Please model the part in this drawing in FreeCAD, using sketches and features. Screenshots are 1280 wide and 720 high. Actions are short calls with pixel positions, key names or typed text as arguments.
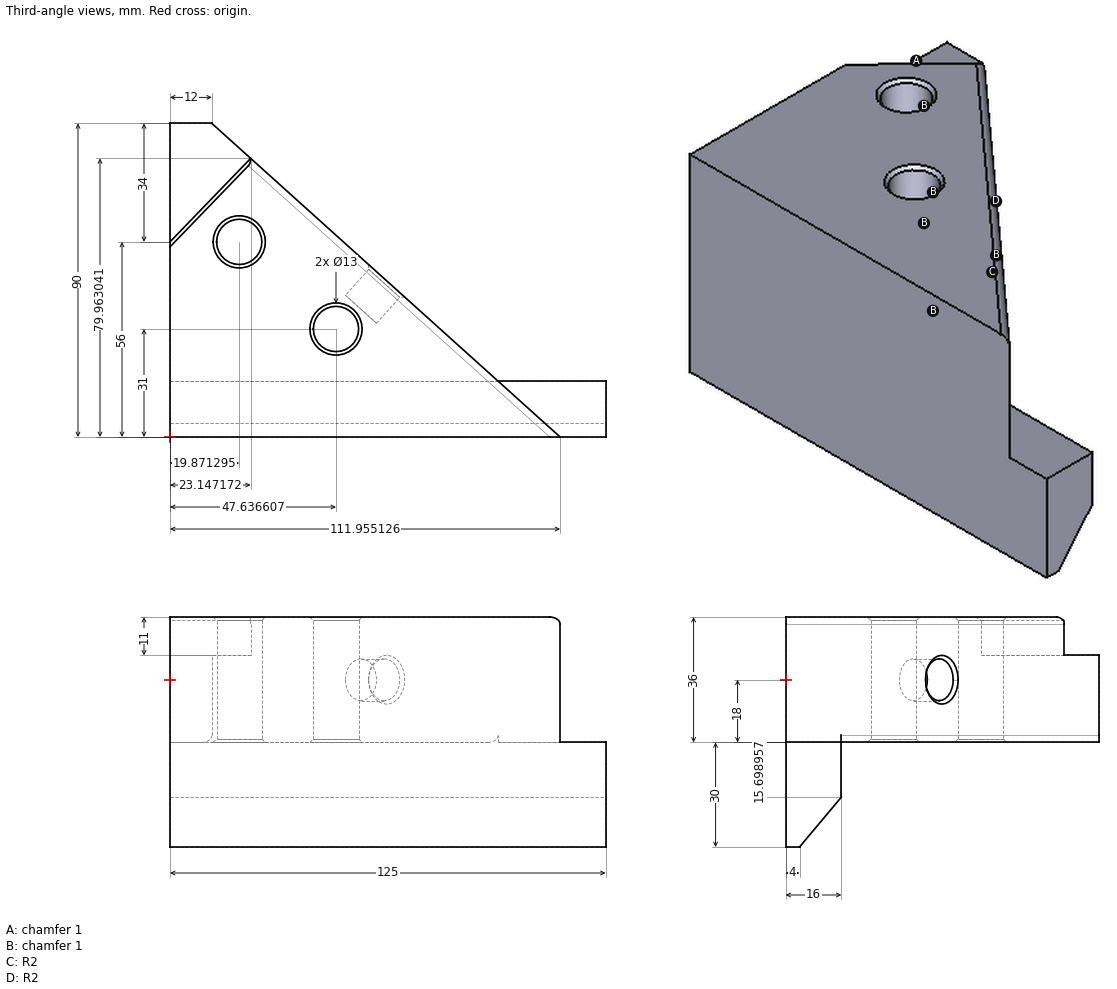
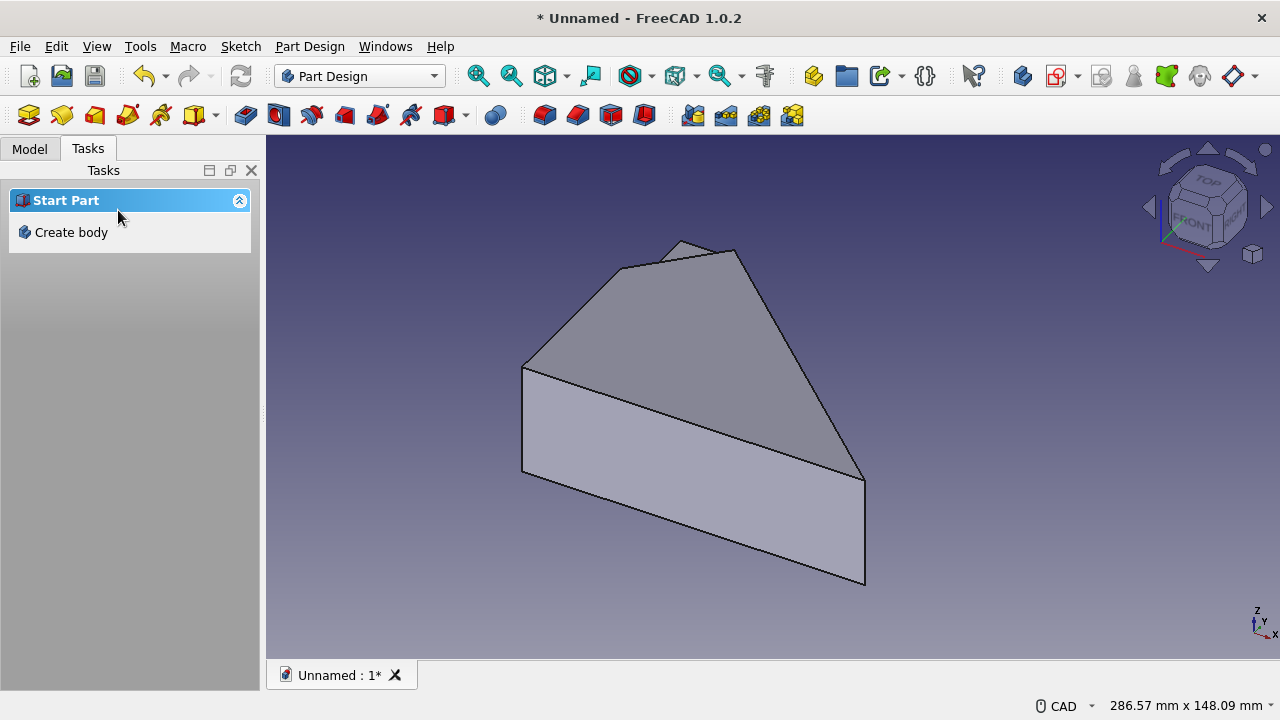
key(4)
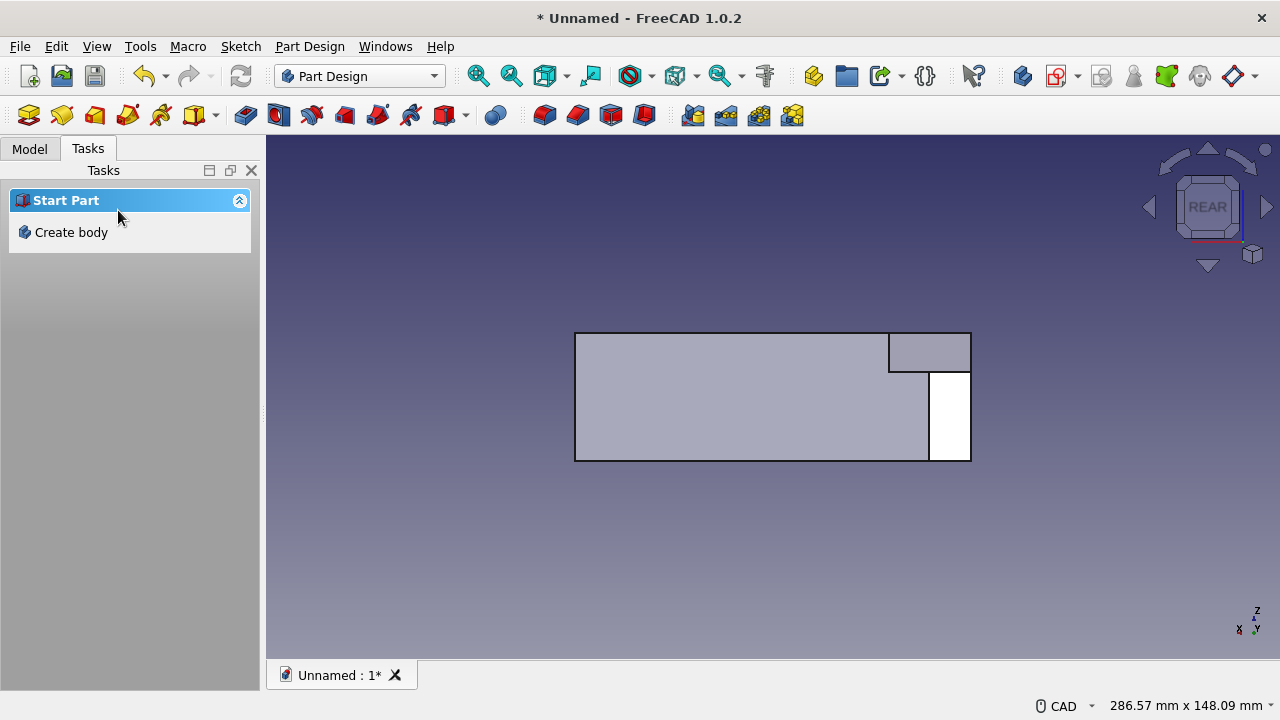
click(479, 76)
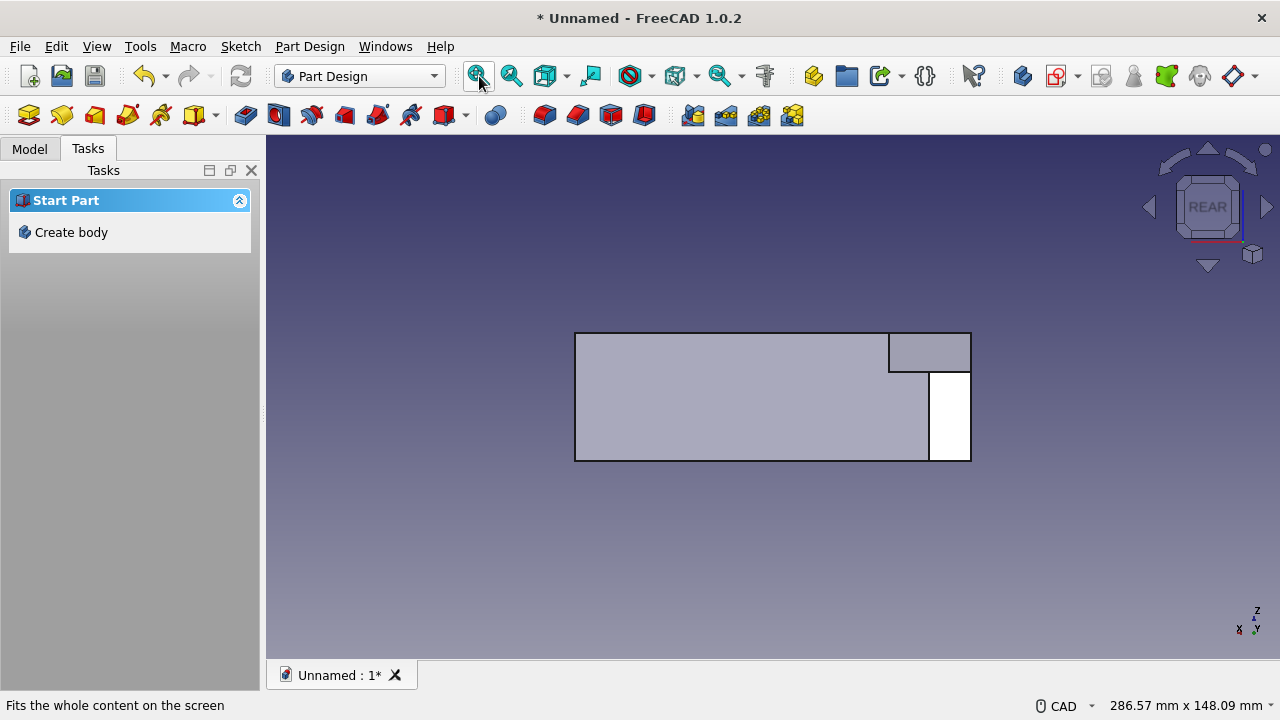
click(651, 396)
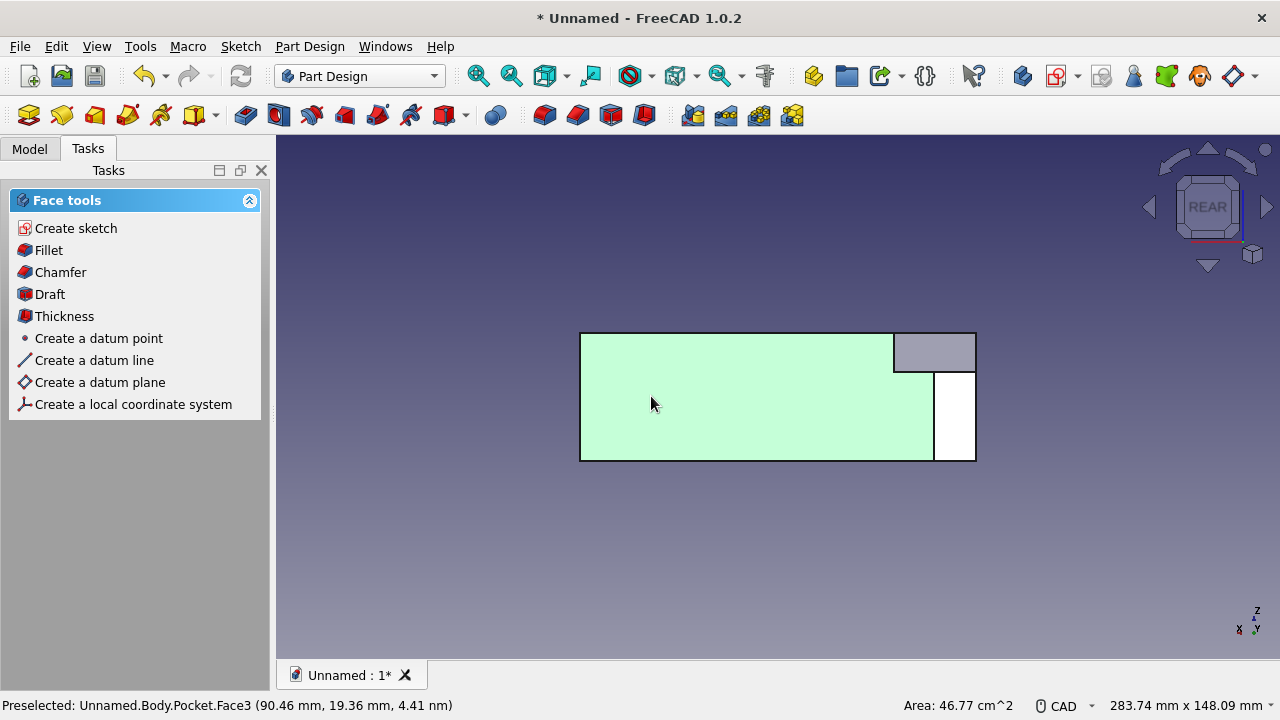
click(1056, 76)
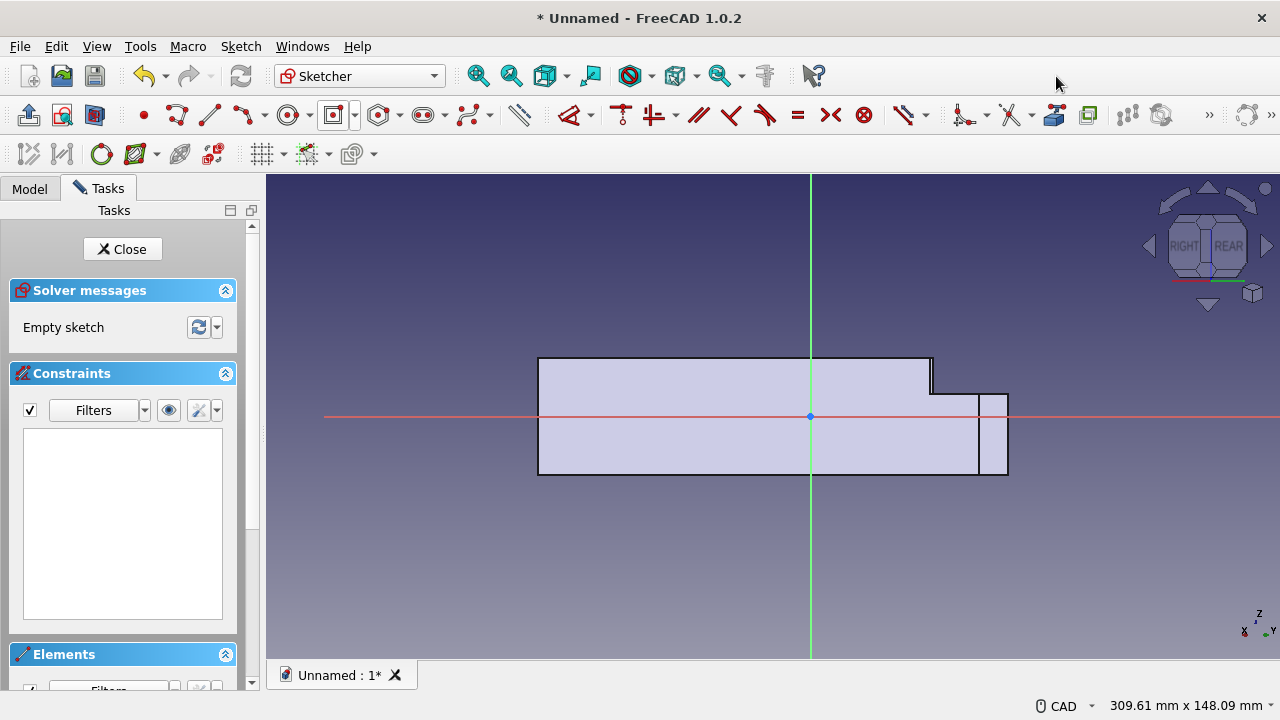
click(95, 116)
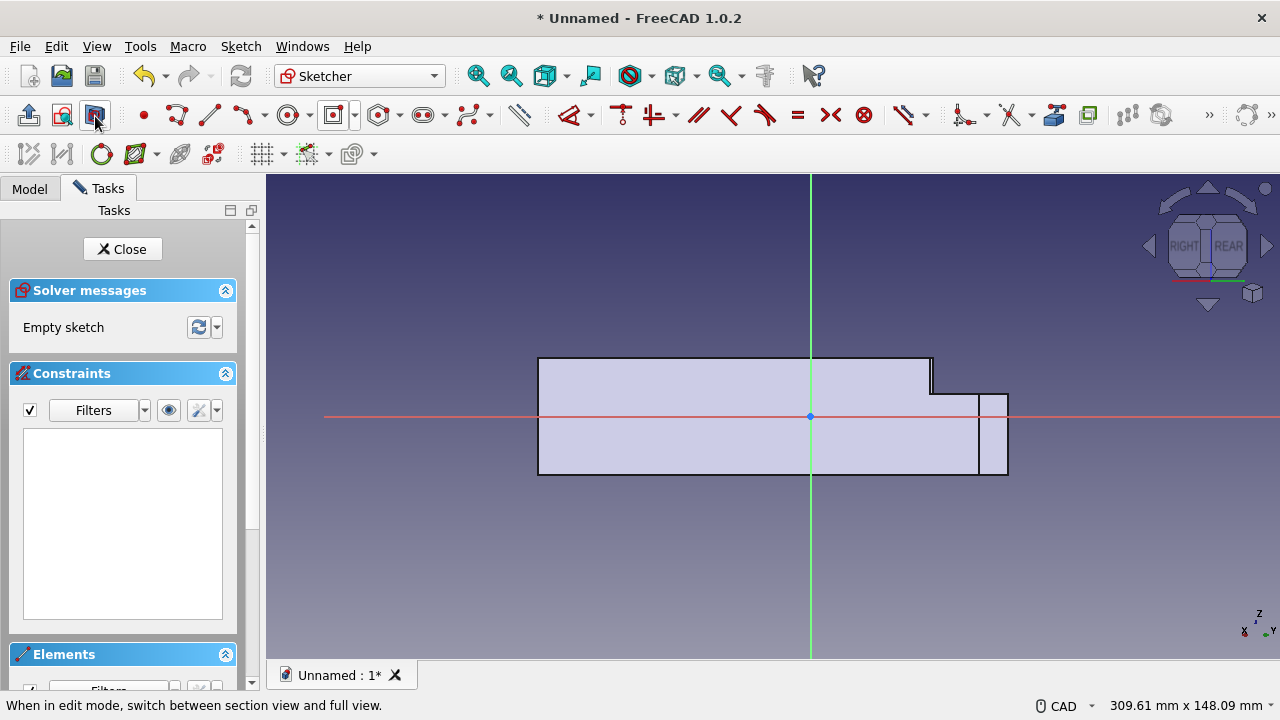
scroll(785, 416, up, 10)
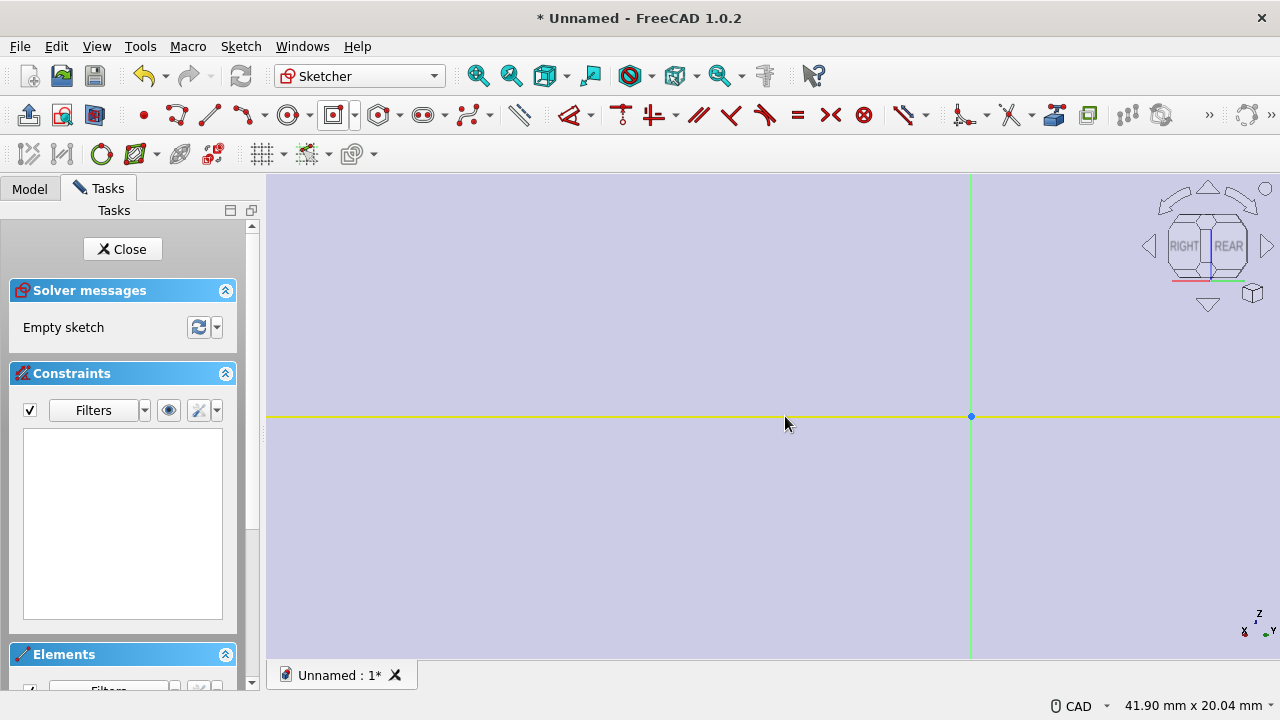
click(288, 116)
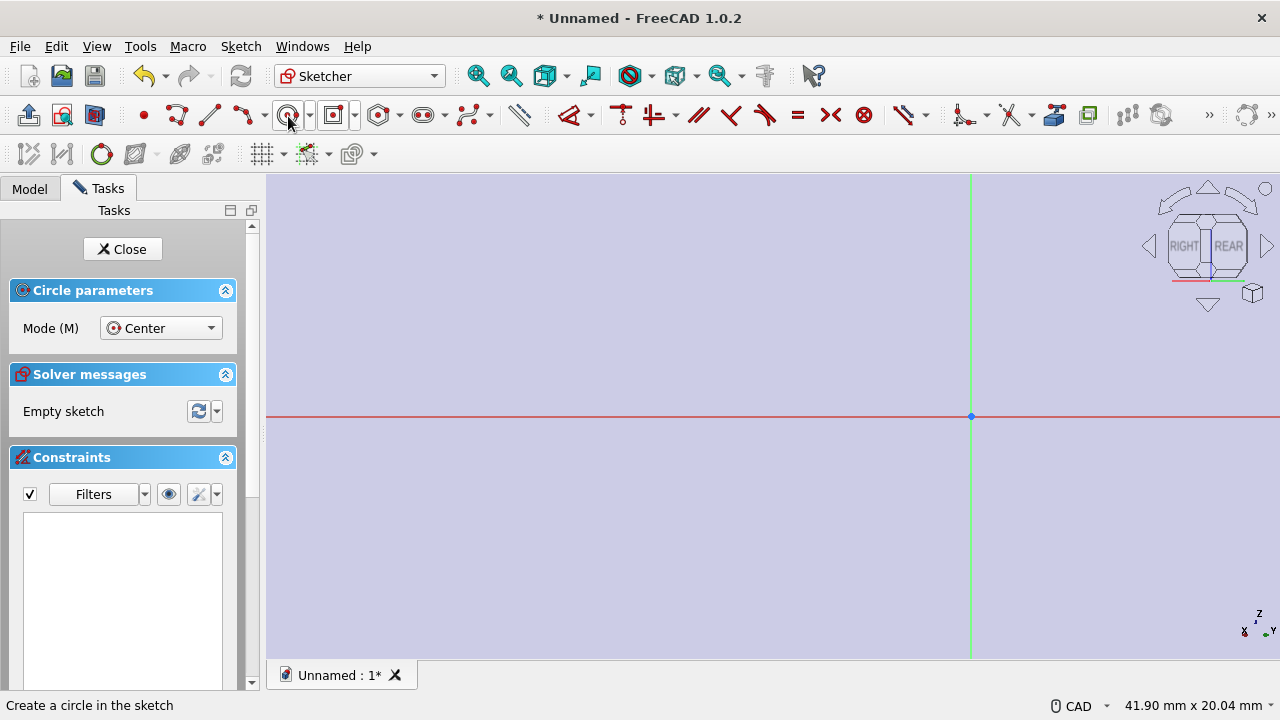
click(579, 416)
click(682, 314)
key(Escape)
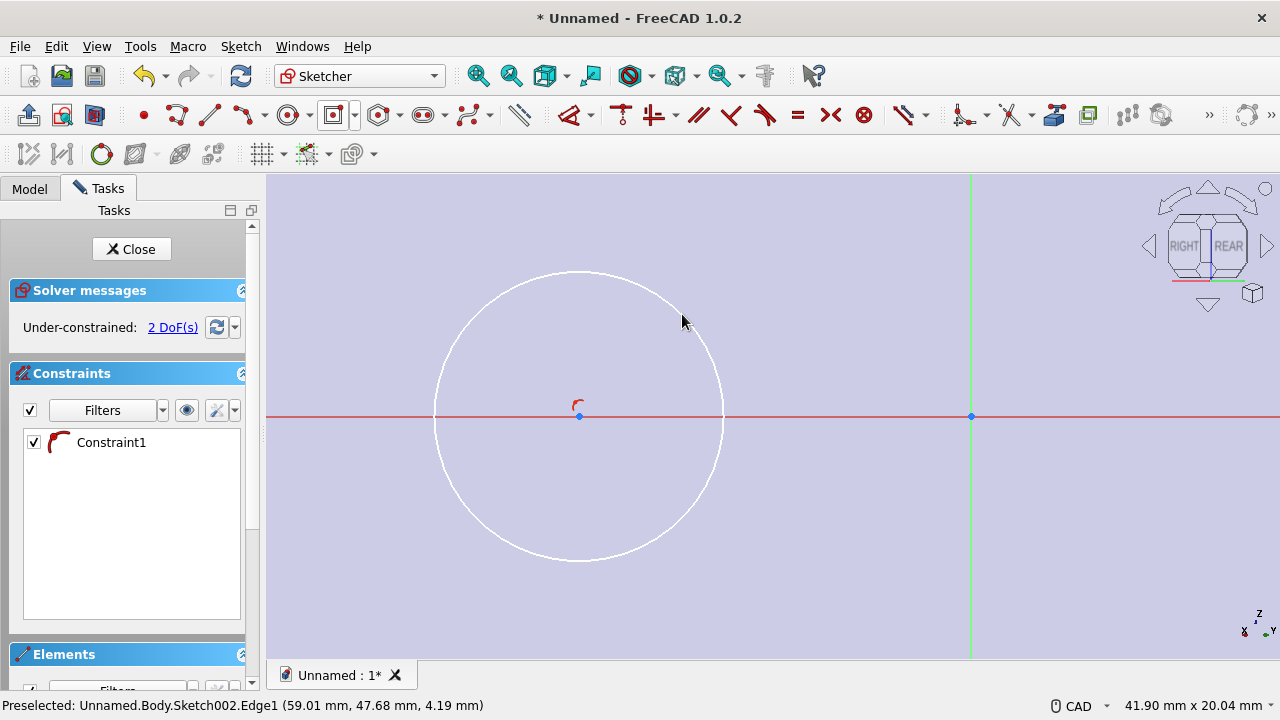
click(568, 116)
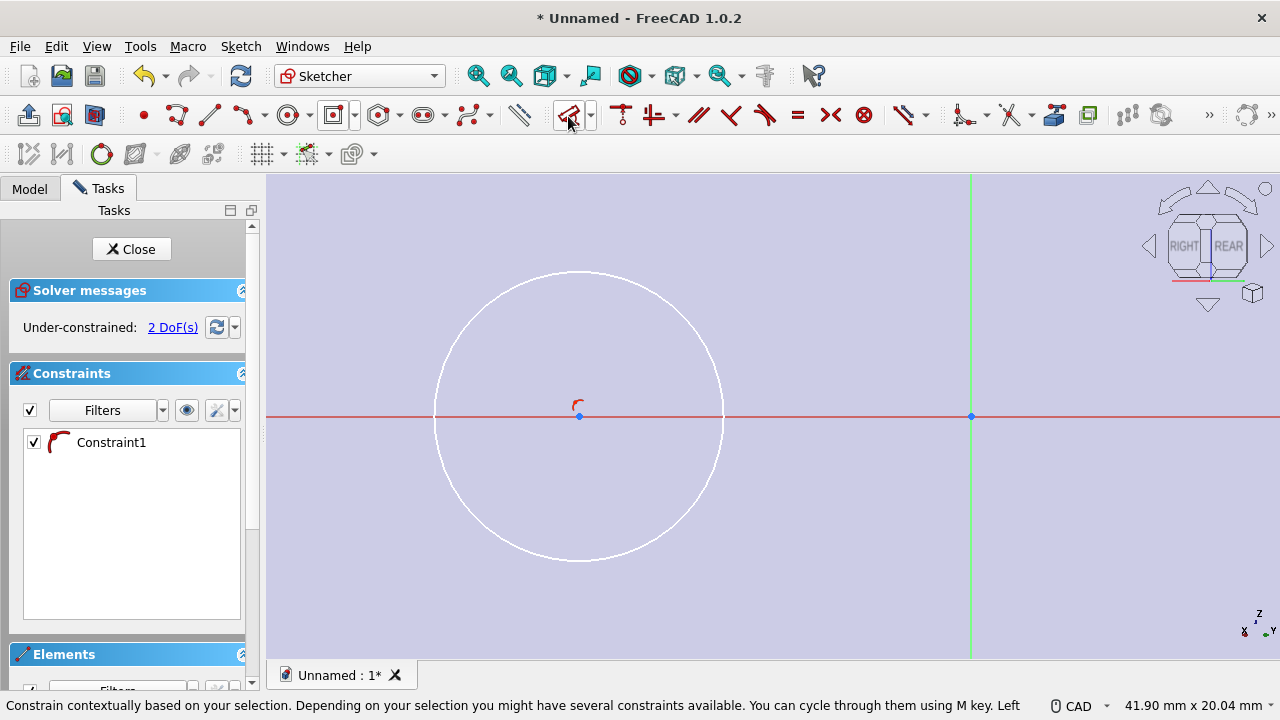
click(681, 314)
click(704, 291)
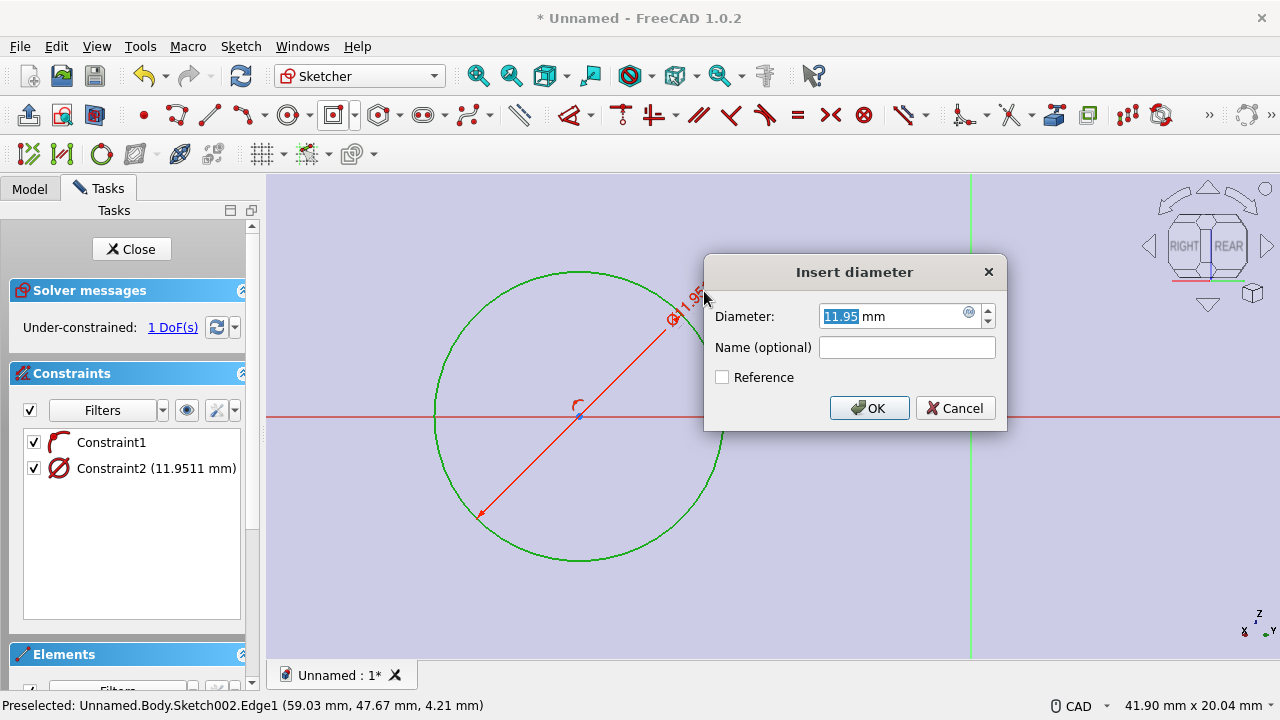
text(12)
key(Return)